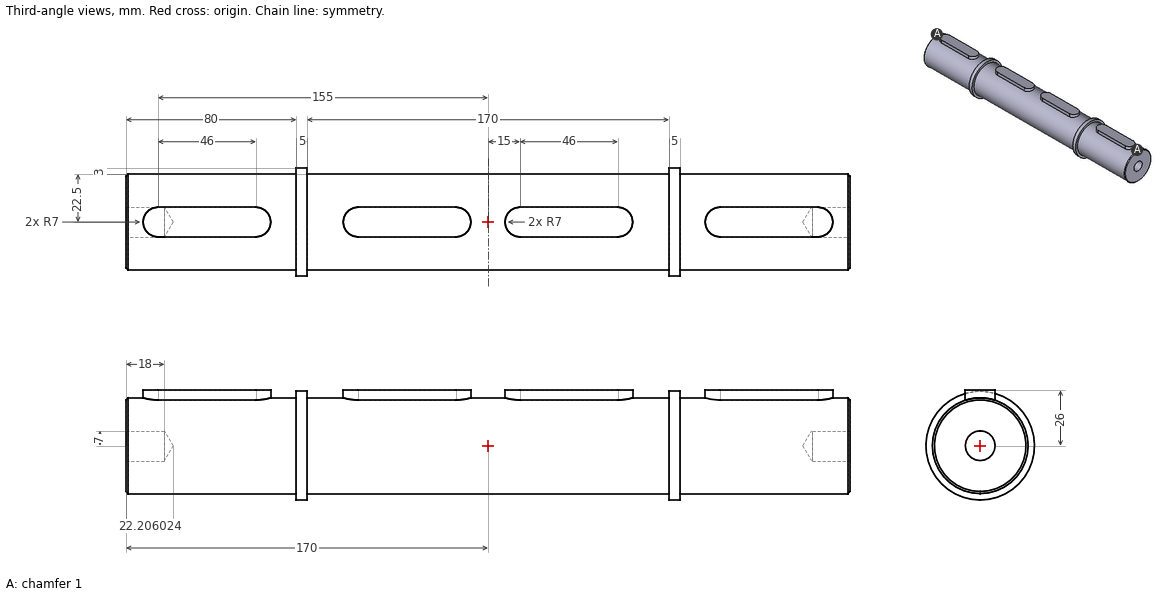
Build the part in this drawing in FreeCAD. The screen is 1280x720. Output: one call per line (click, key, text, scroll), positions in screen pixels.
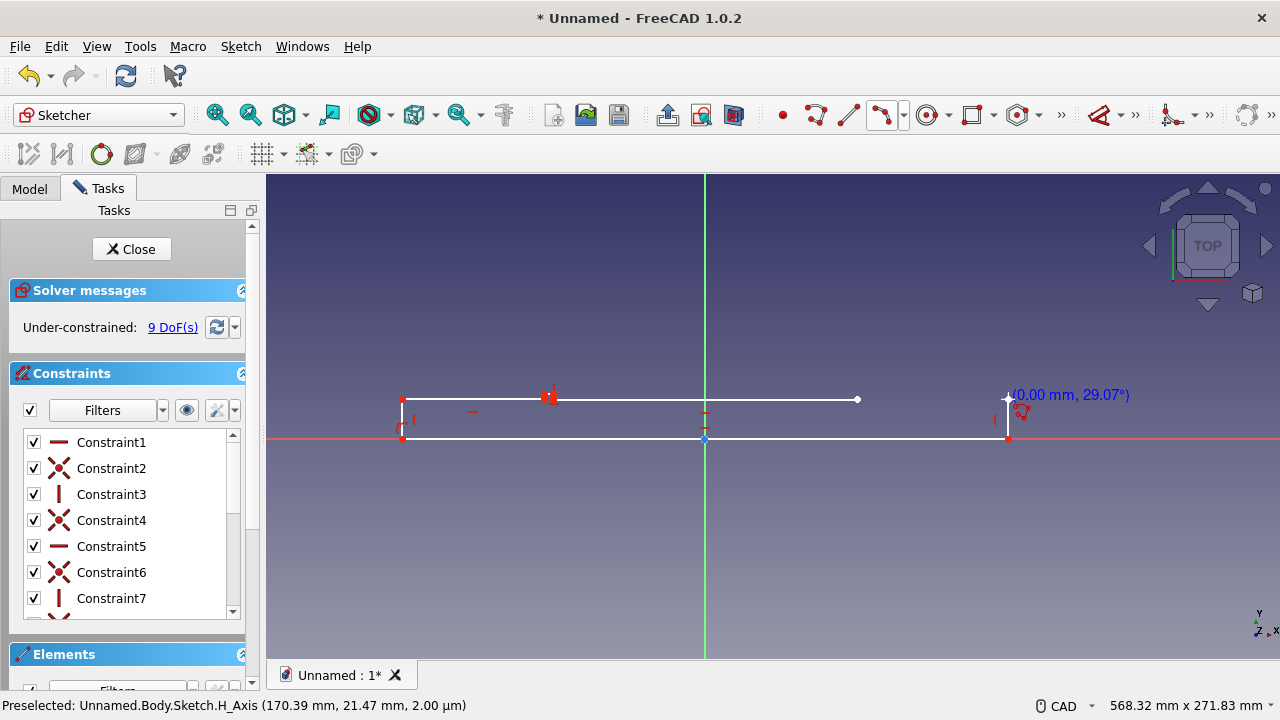
scroll(866, 399, up, 3)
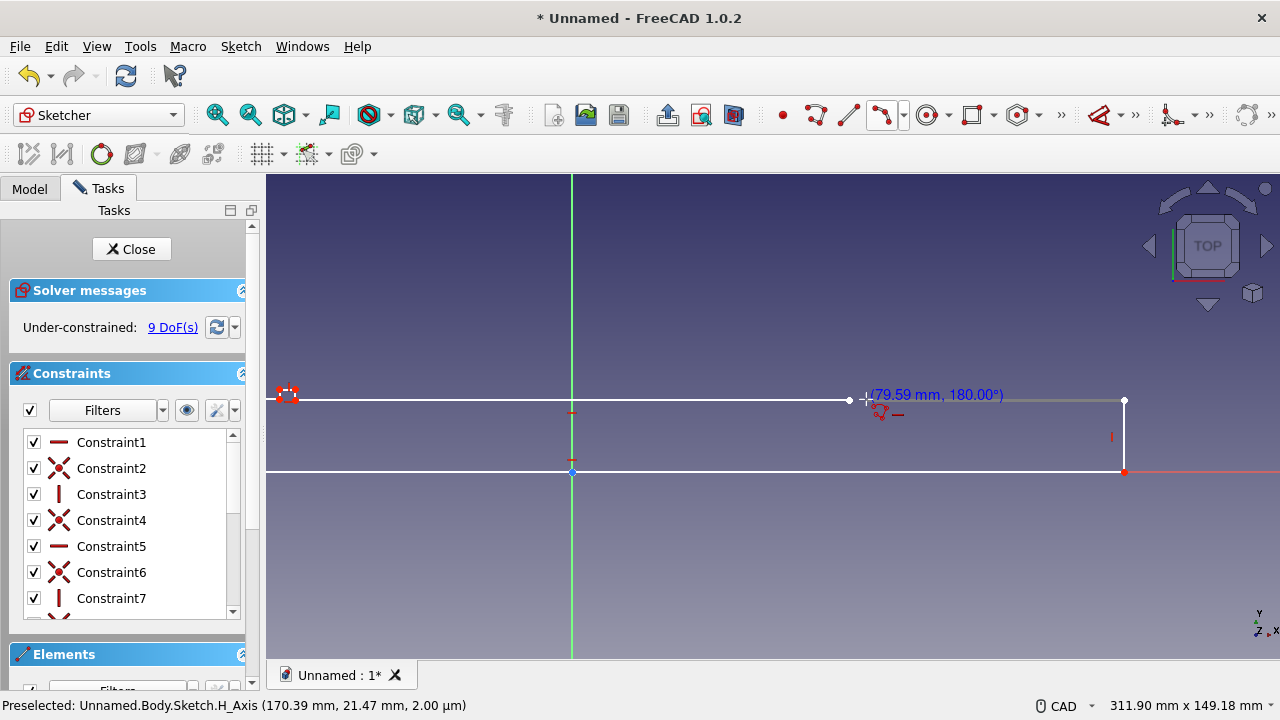
click(865, 399)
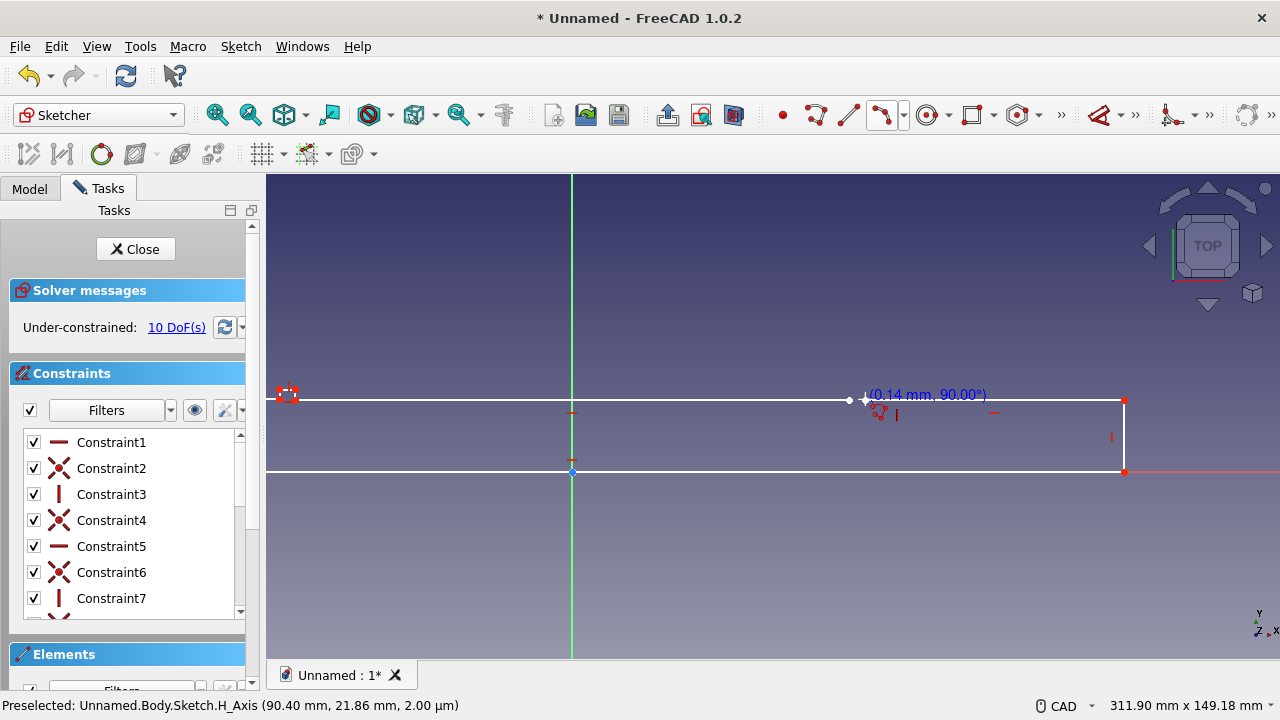
scroll(865, 389, up, 3)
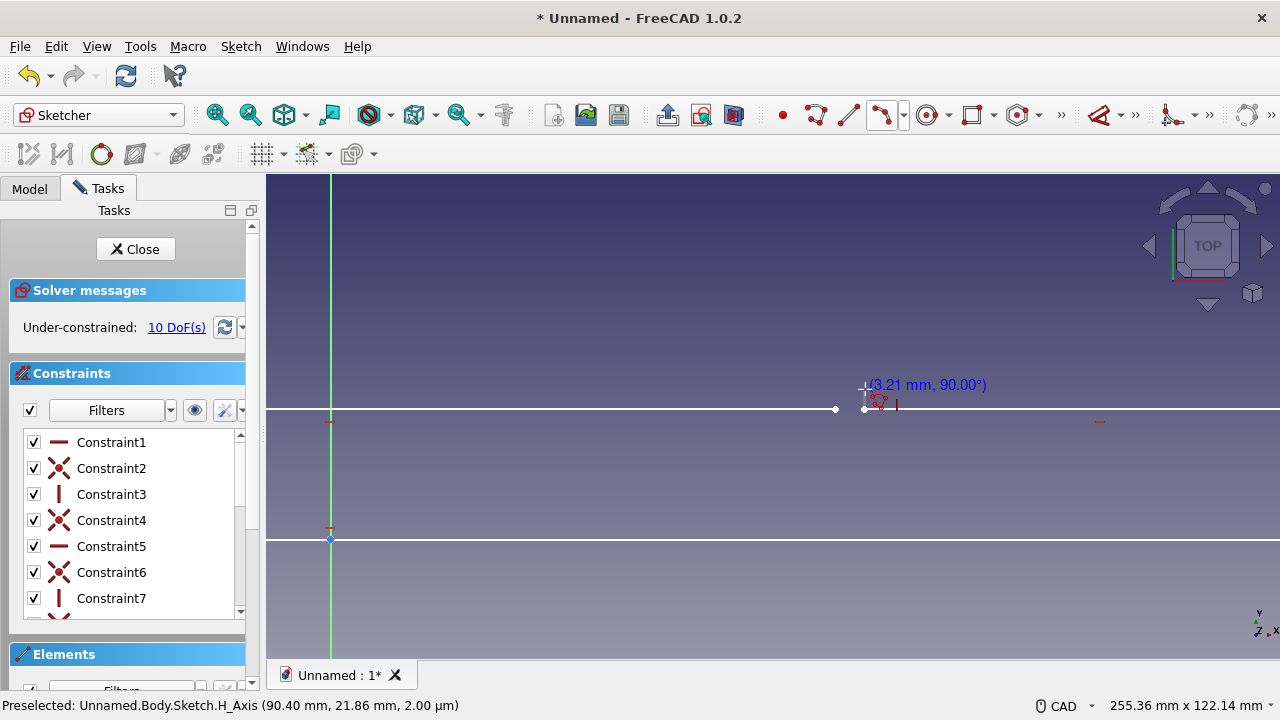
click(865, 389)
click(834, 389)
click(836, 409)
key(Escape)
key(Escape)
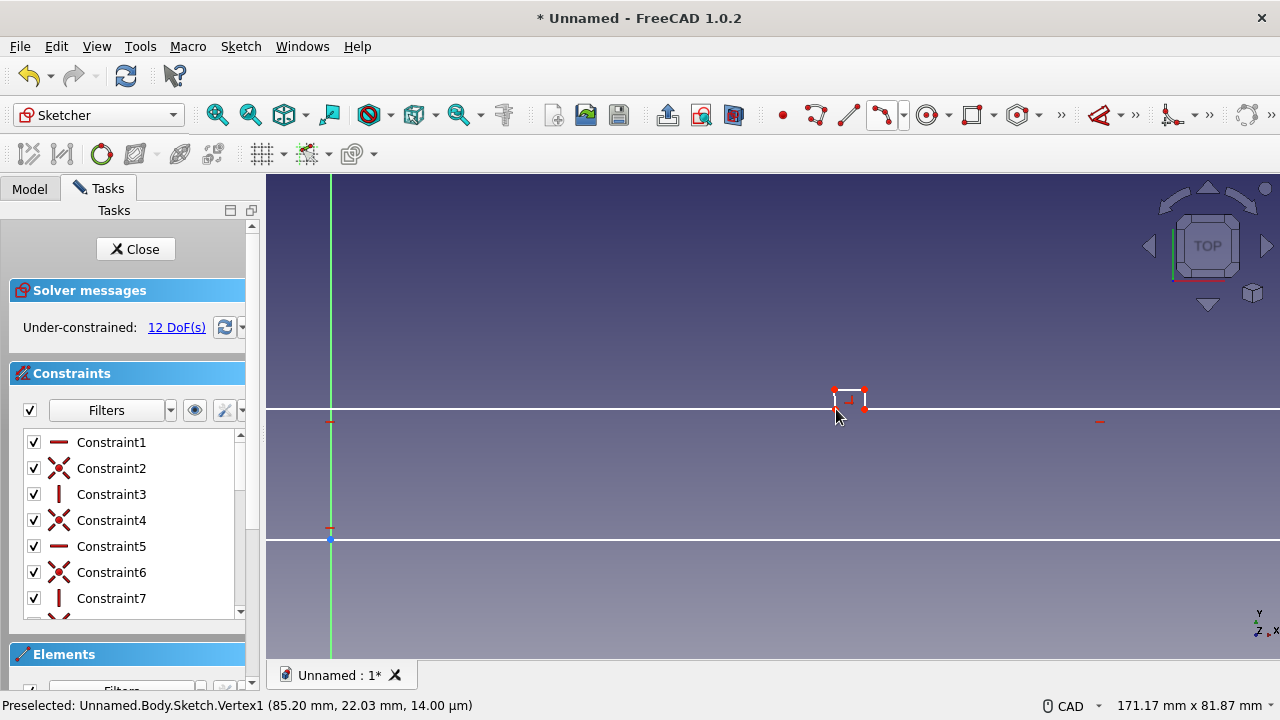
scroll(835, 400, up, 2)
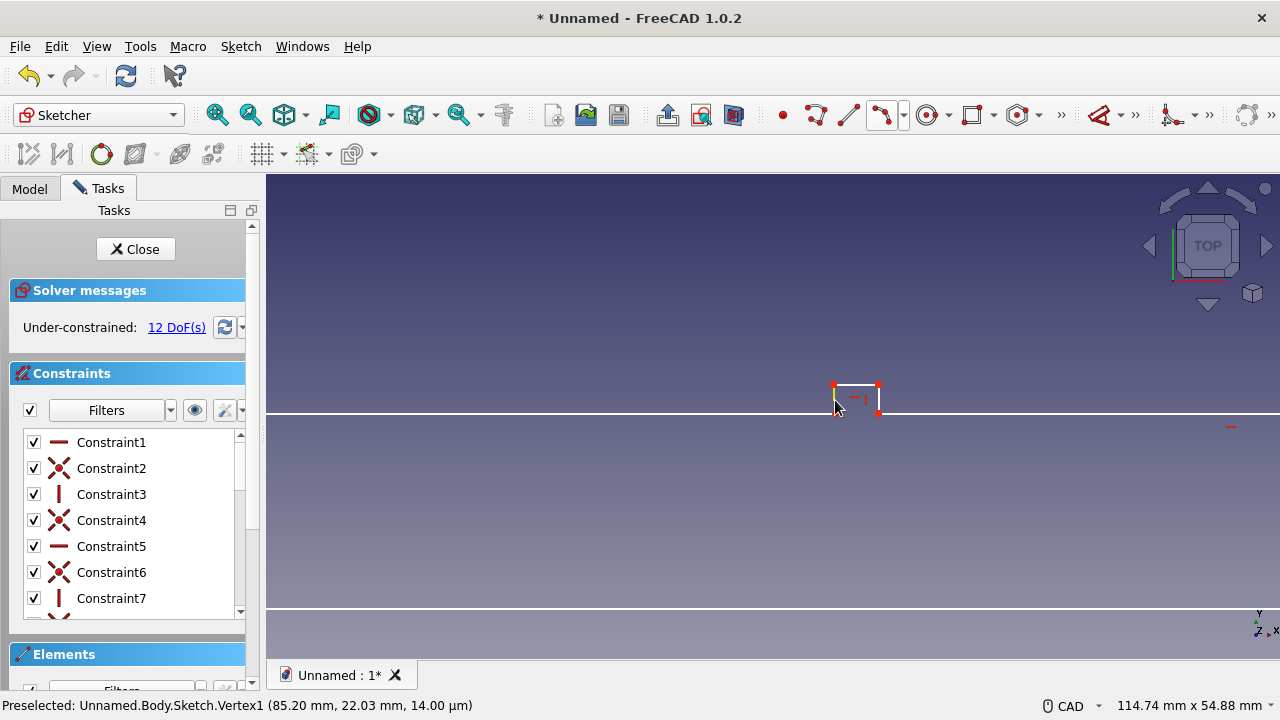
click(834, 399)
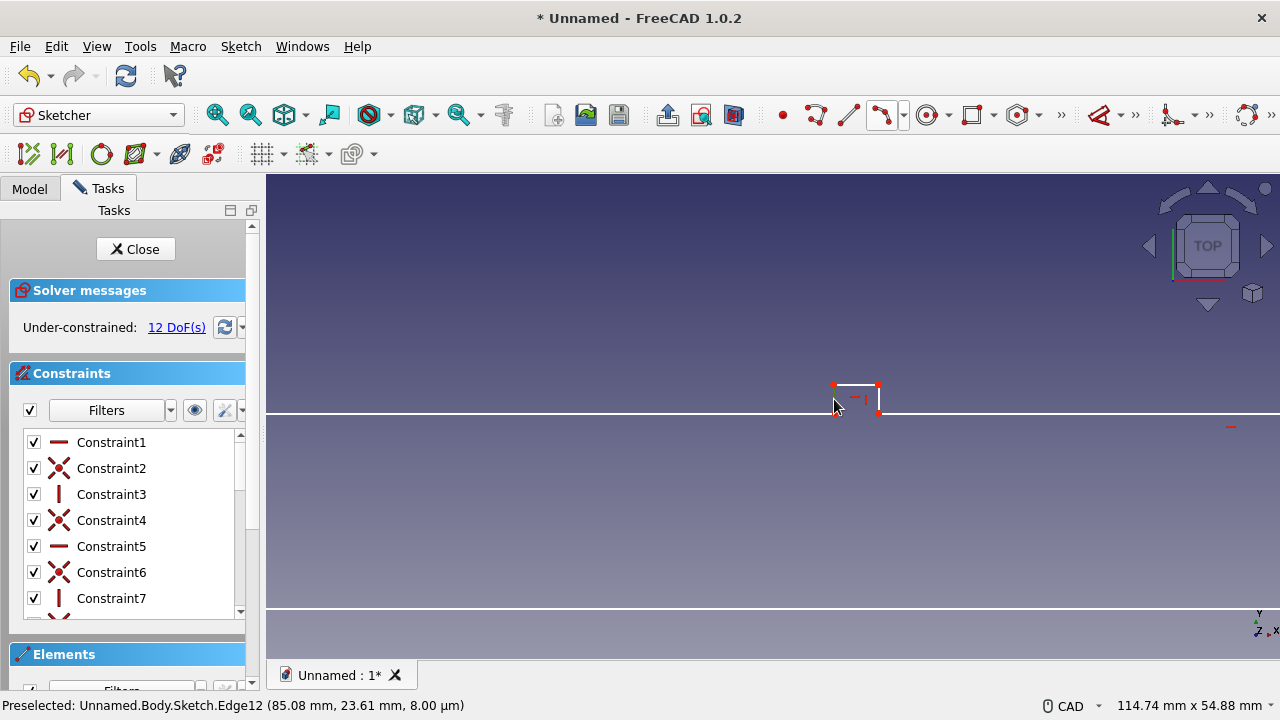
key(v)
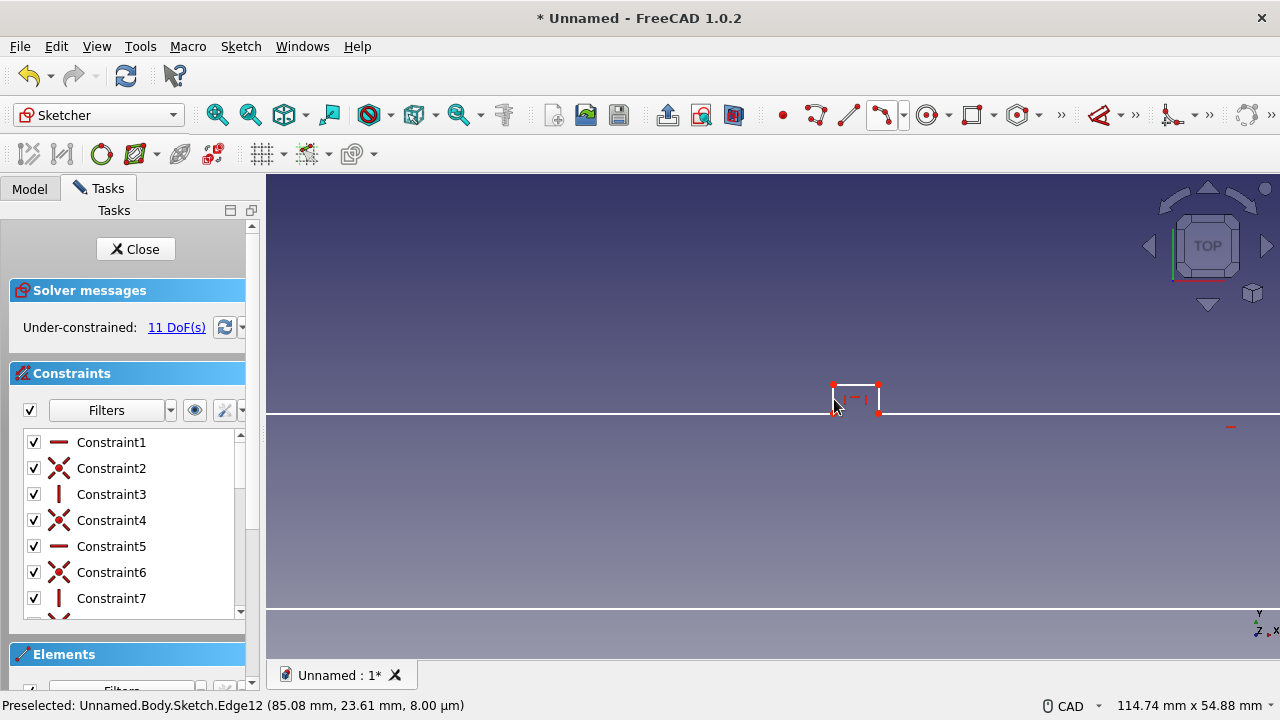
scroll(862, 396, down, 8)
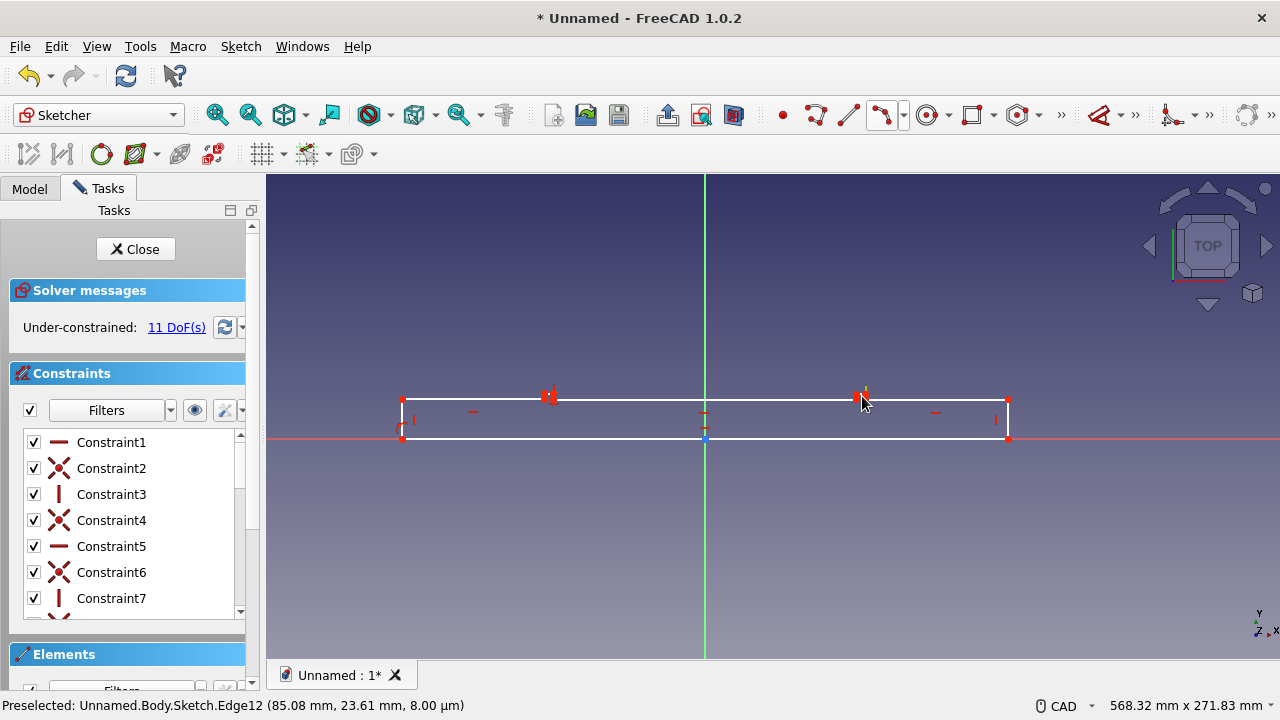
click(402, 399)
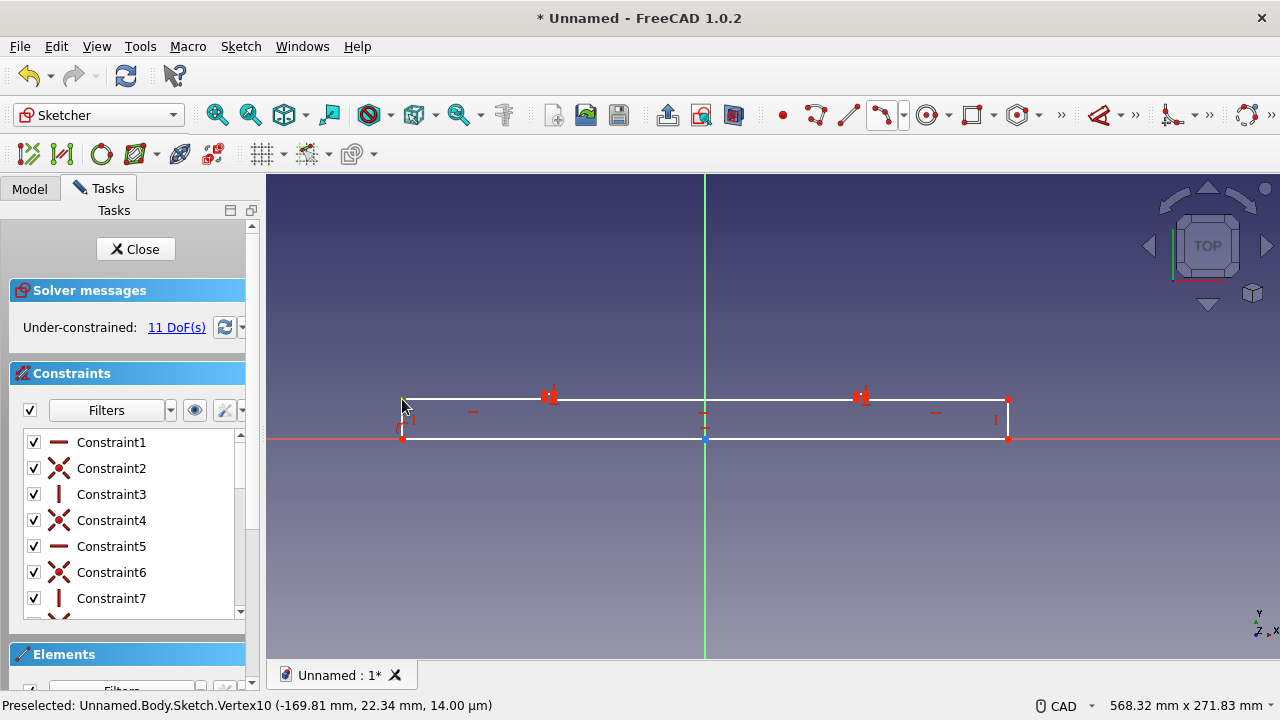
click(1008, 400)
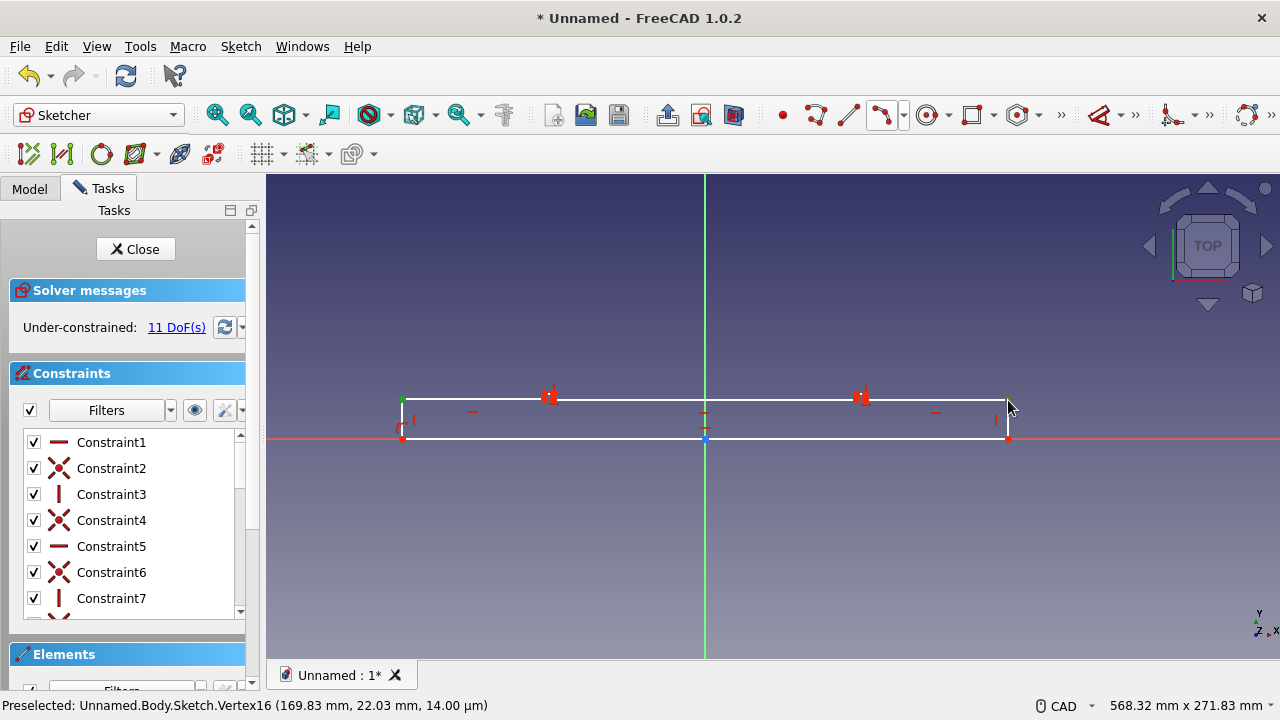
click(705, 600)